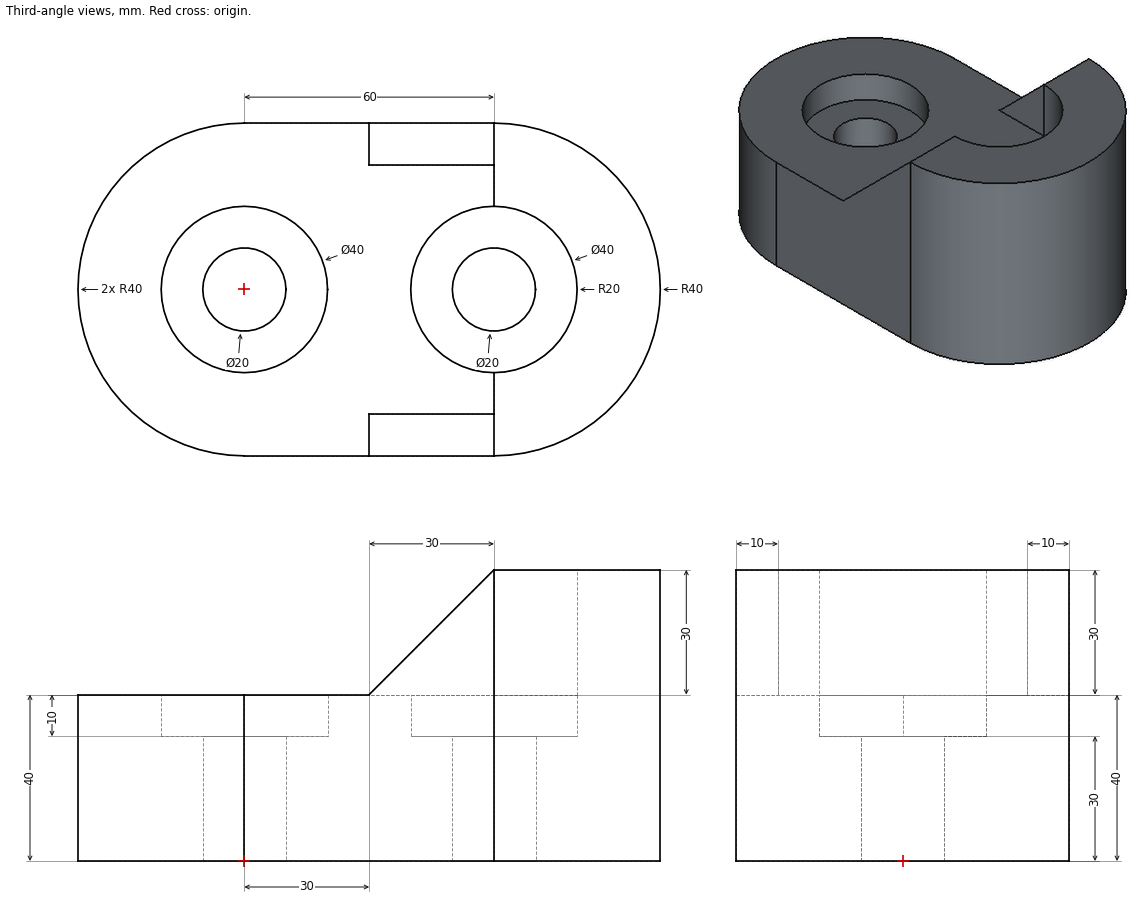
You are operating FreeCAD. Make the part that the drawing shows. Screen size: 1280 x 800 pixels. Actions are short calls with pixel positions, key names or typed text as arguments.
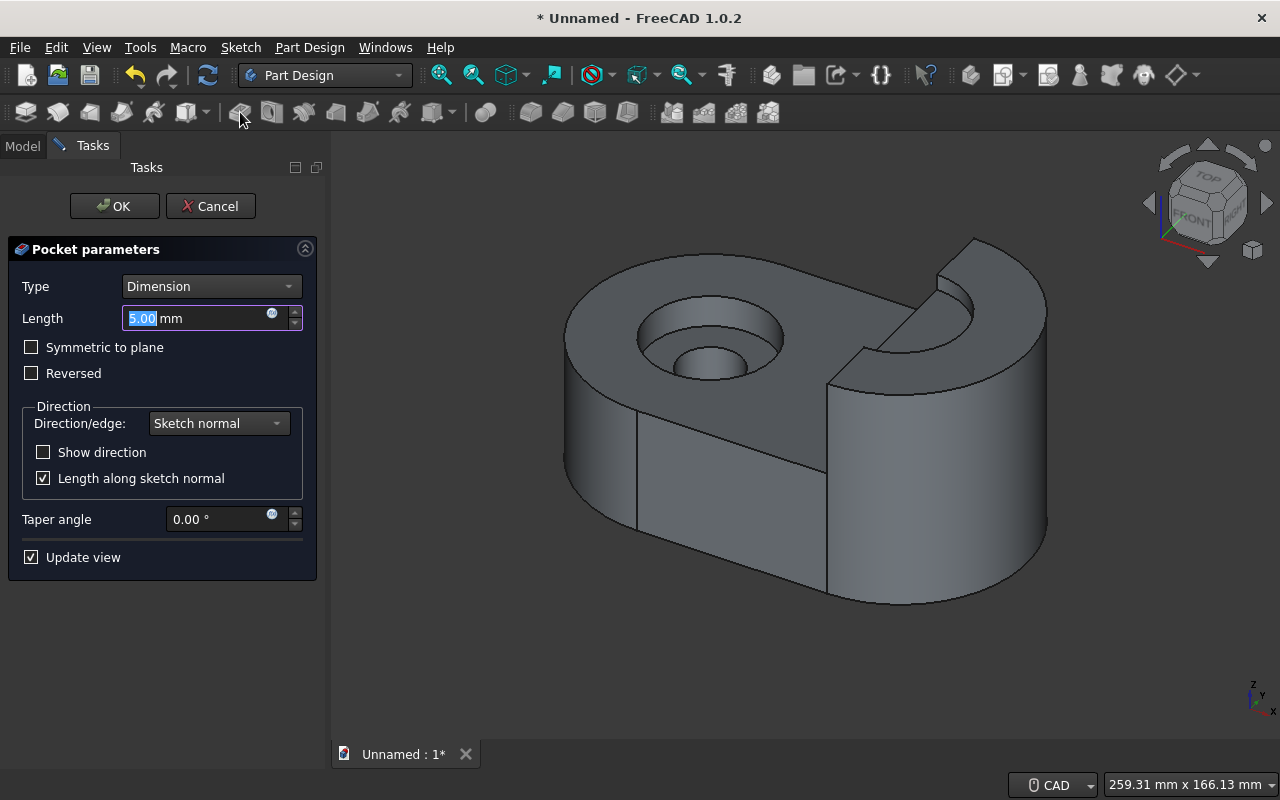
text(30)
key(Tab)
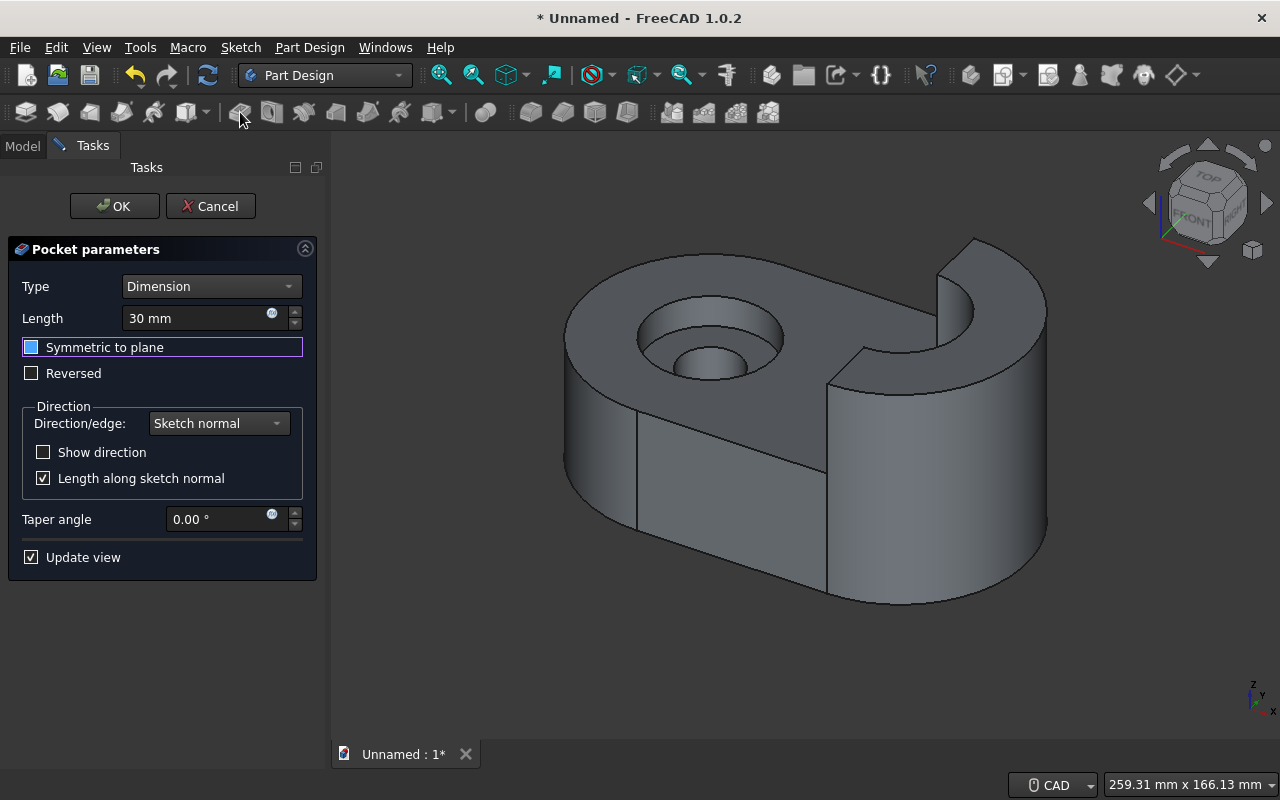
click(115, 206)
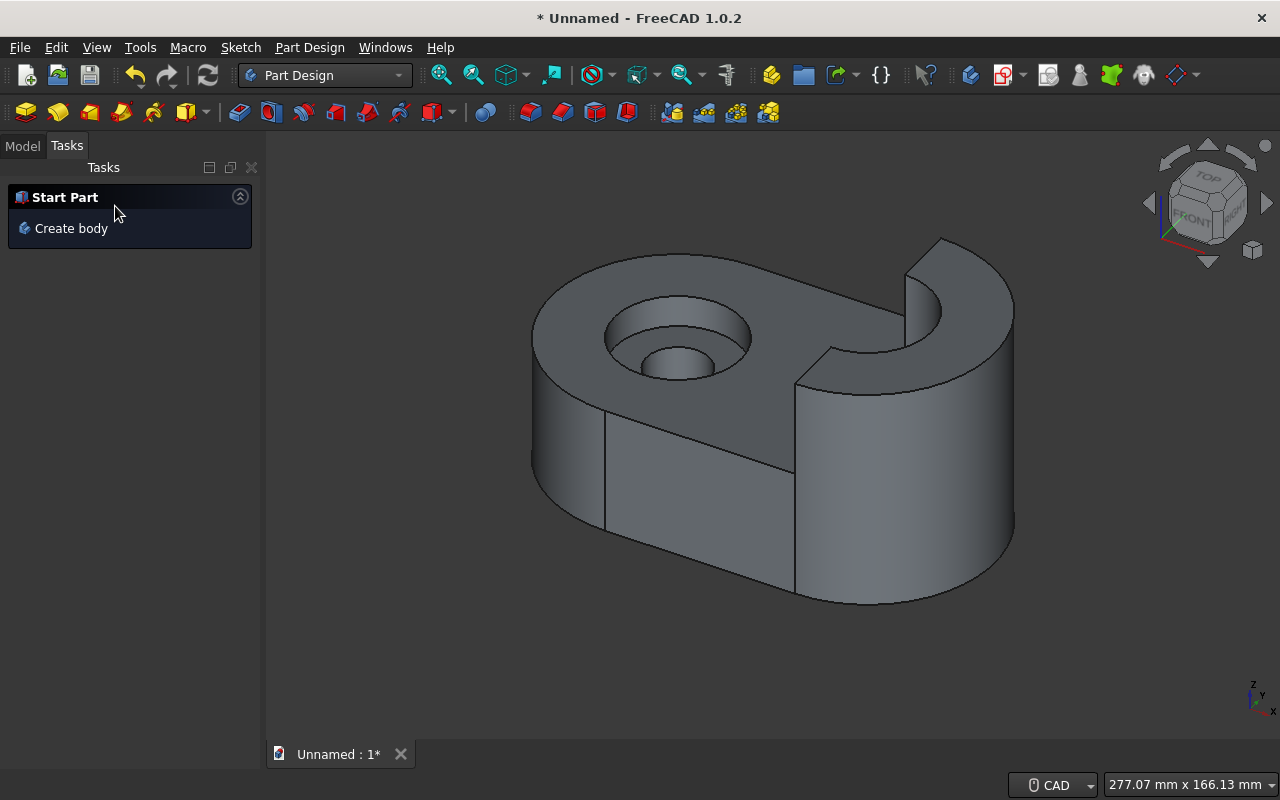
click(775, 397)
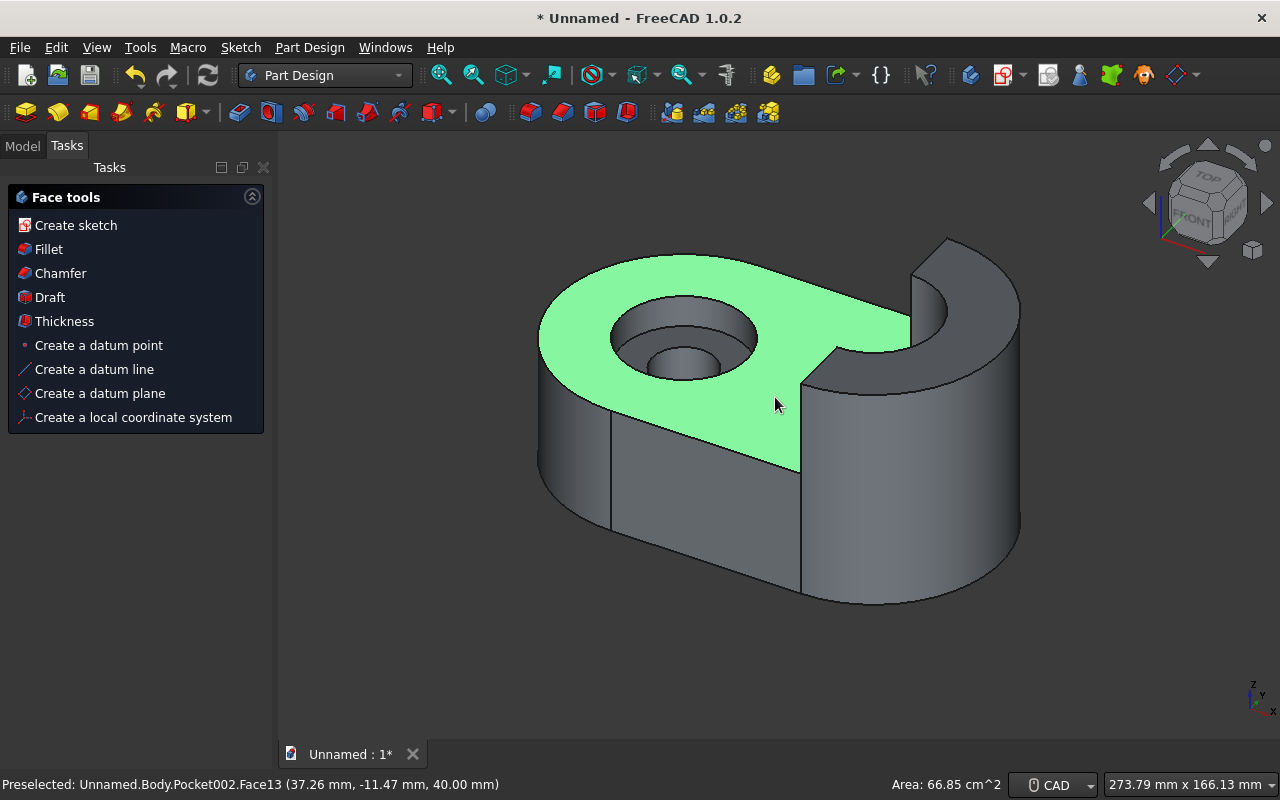
click(1004, 76)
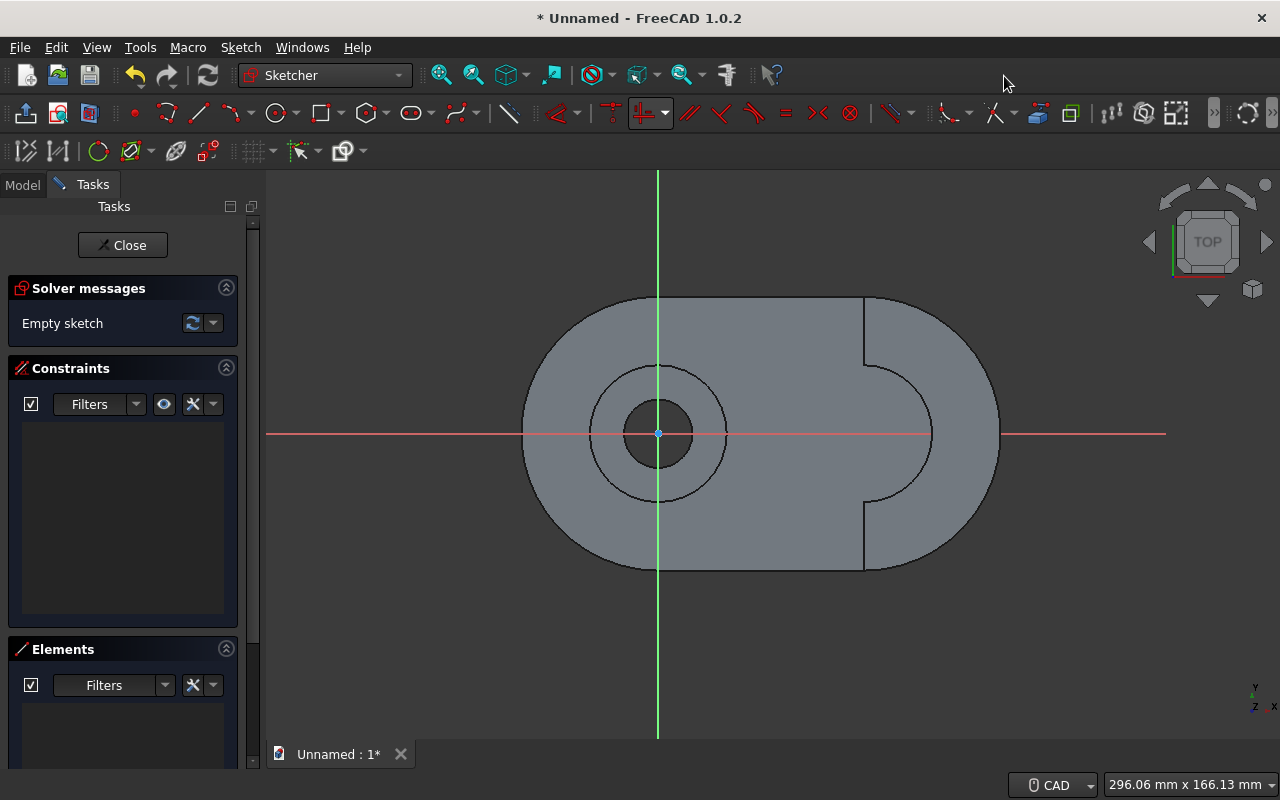
scroll(869, 417, up, 4)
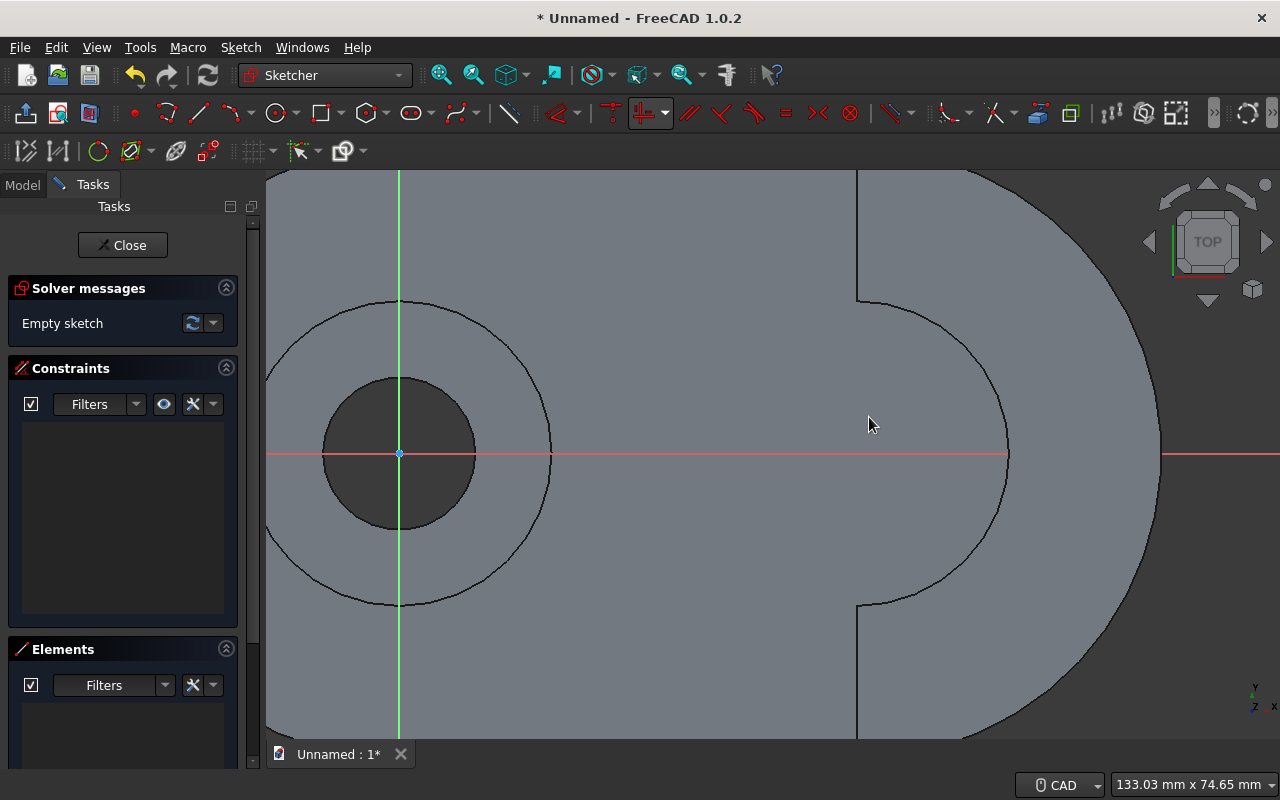
click(276, 114)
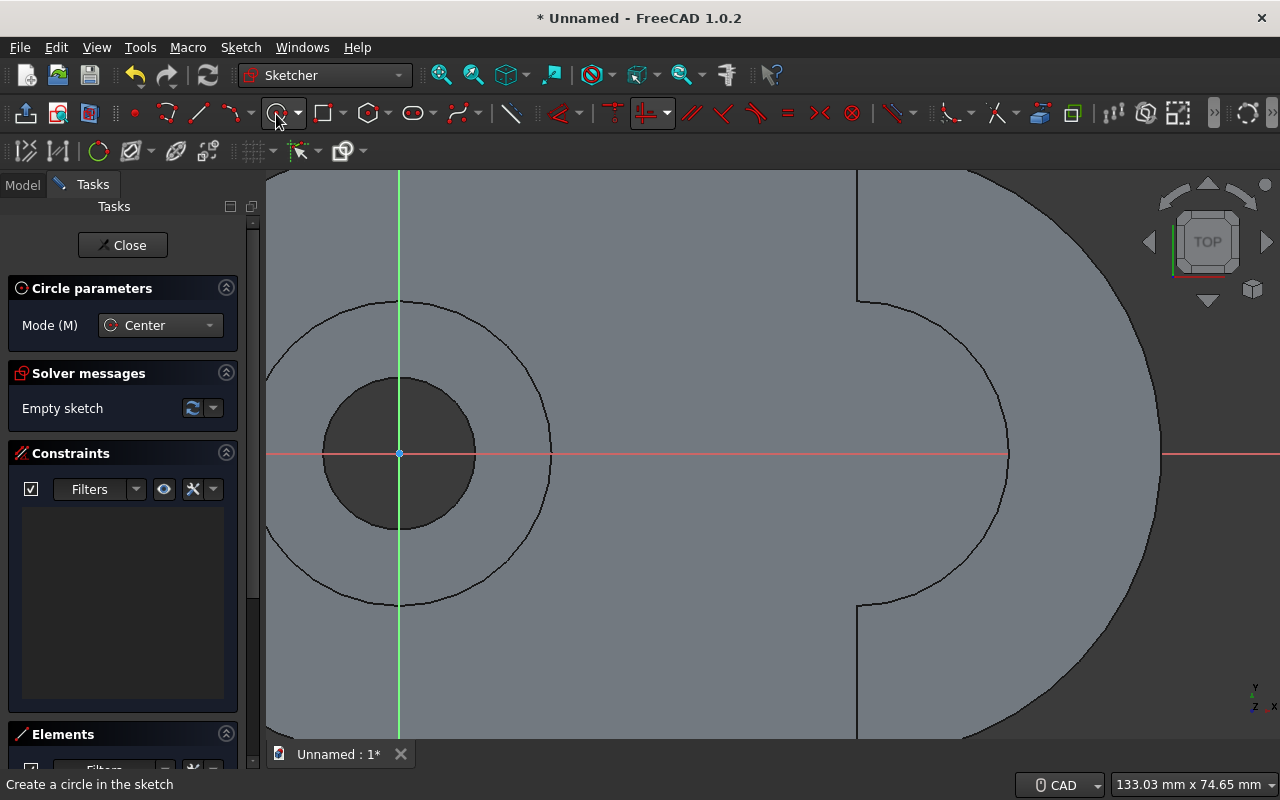
click(857, 454)
move(964, 346)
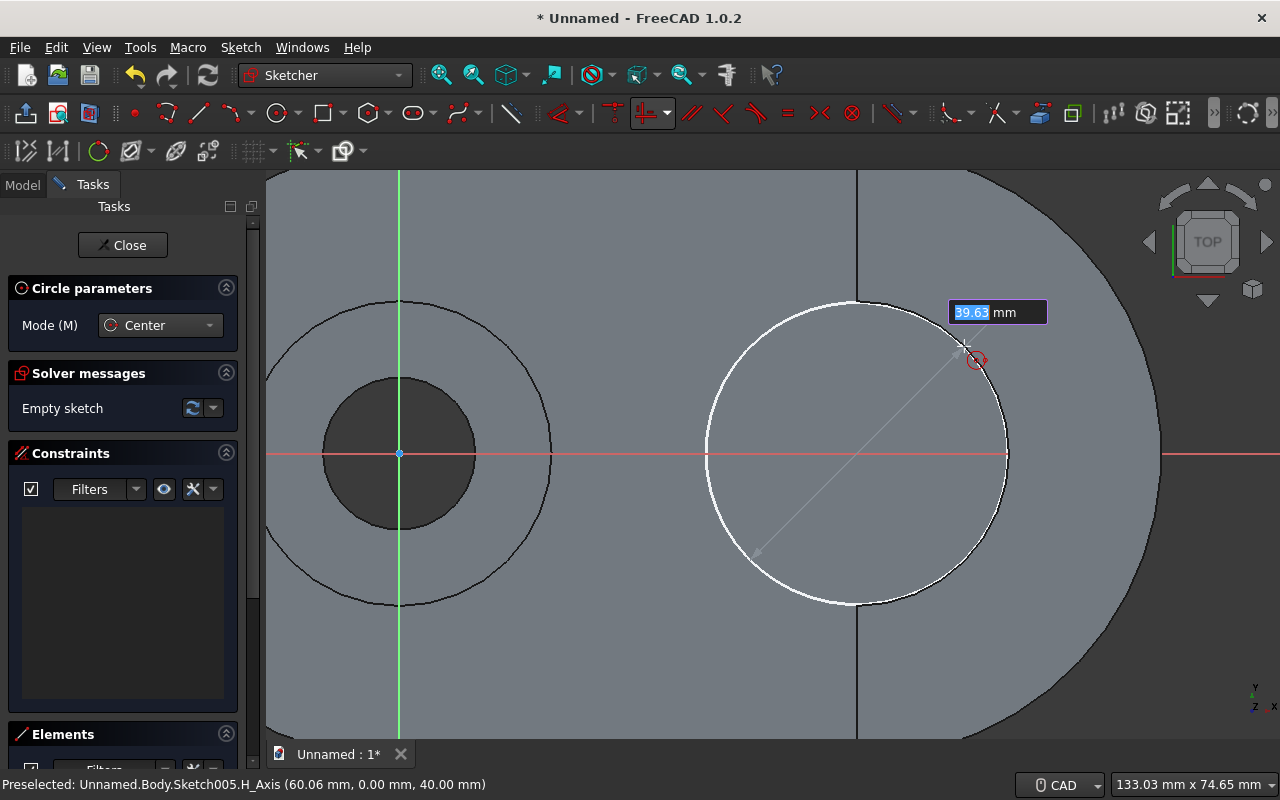
text(40)
key(Return)
key(Escape)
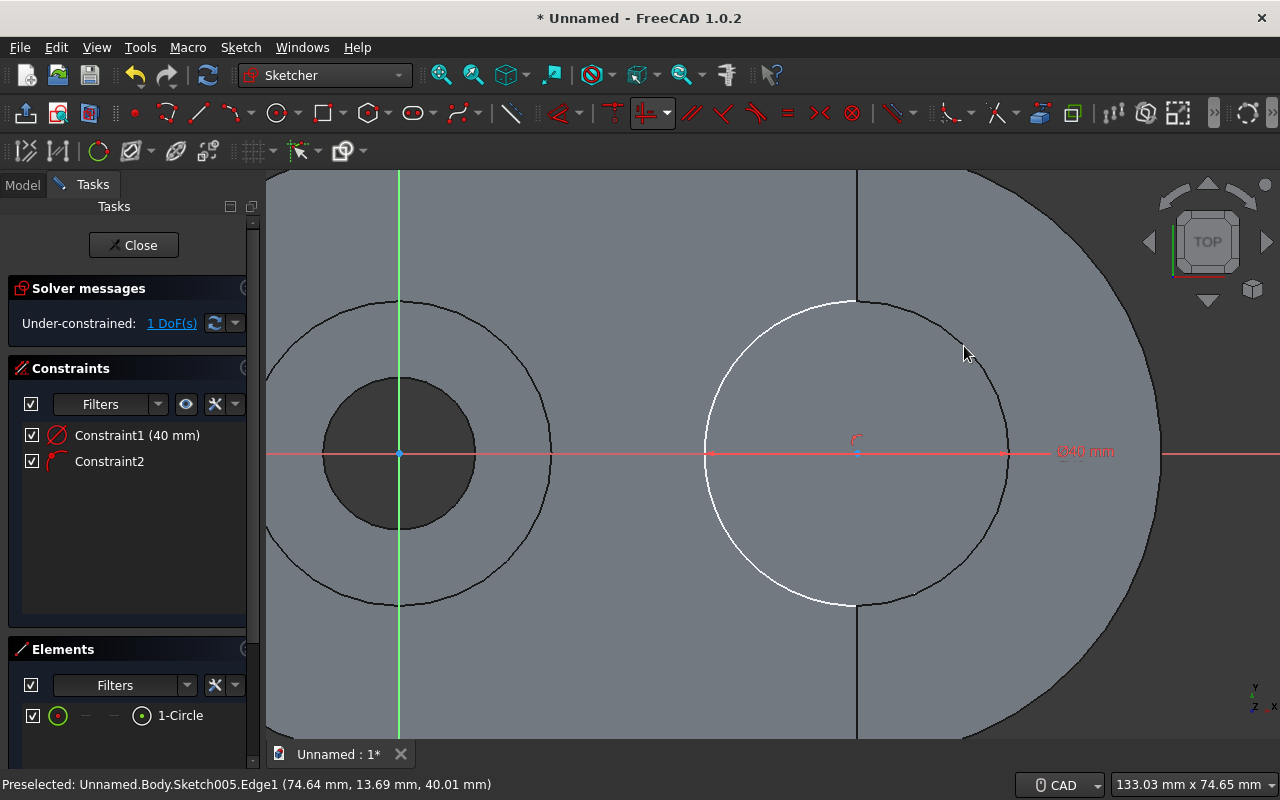
click(558, 114)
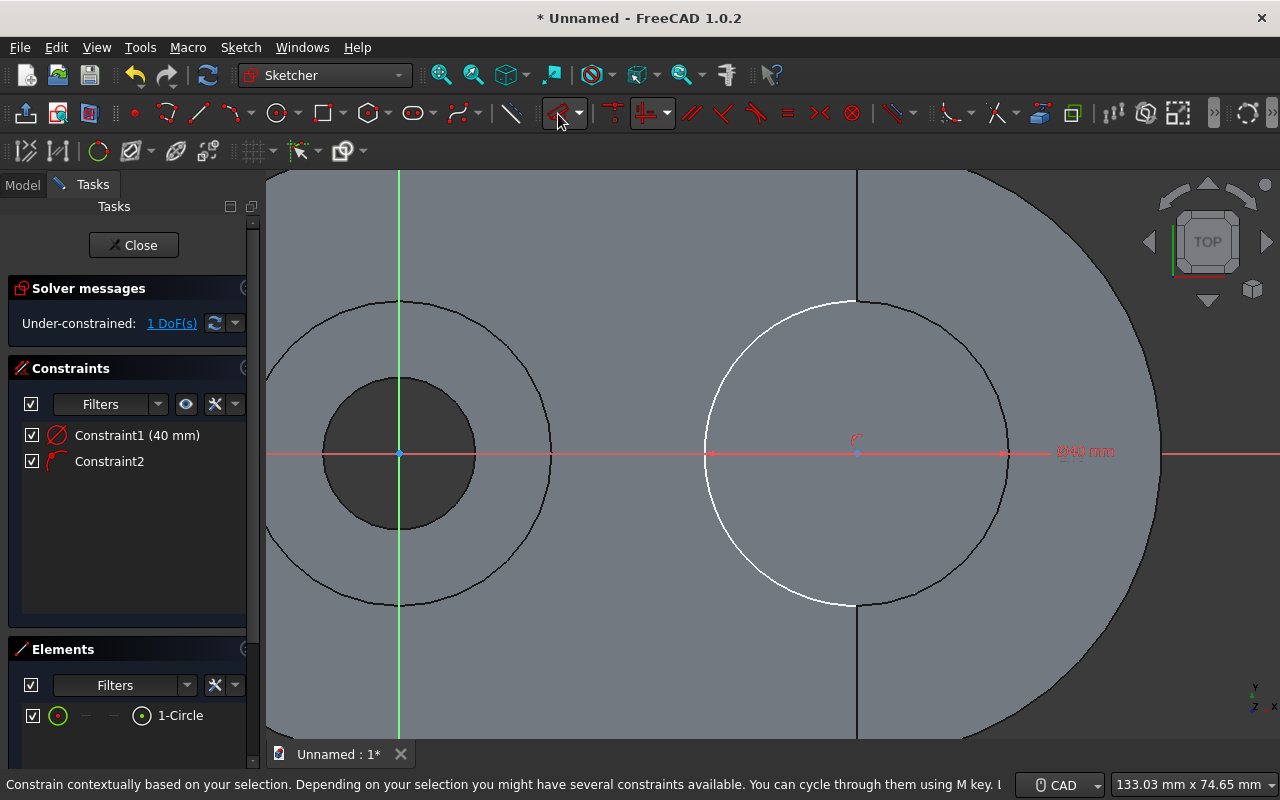
click(857, 454)
click(628, 488)